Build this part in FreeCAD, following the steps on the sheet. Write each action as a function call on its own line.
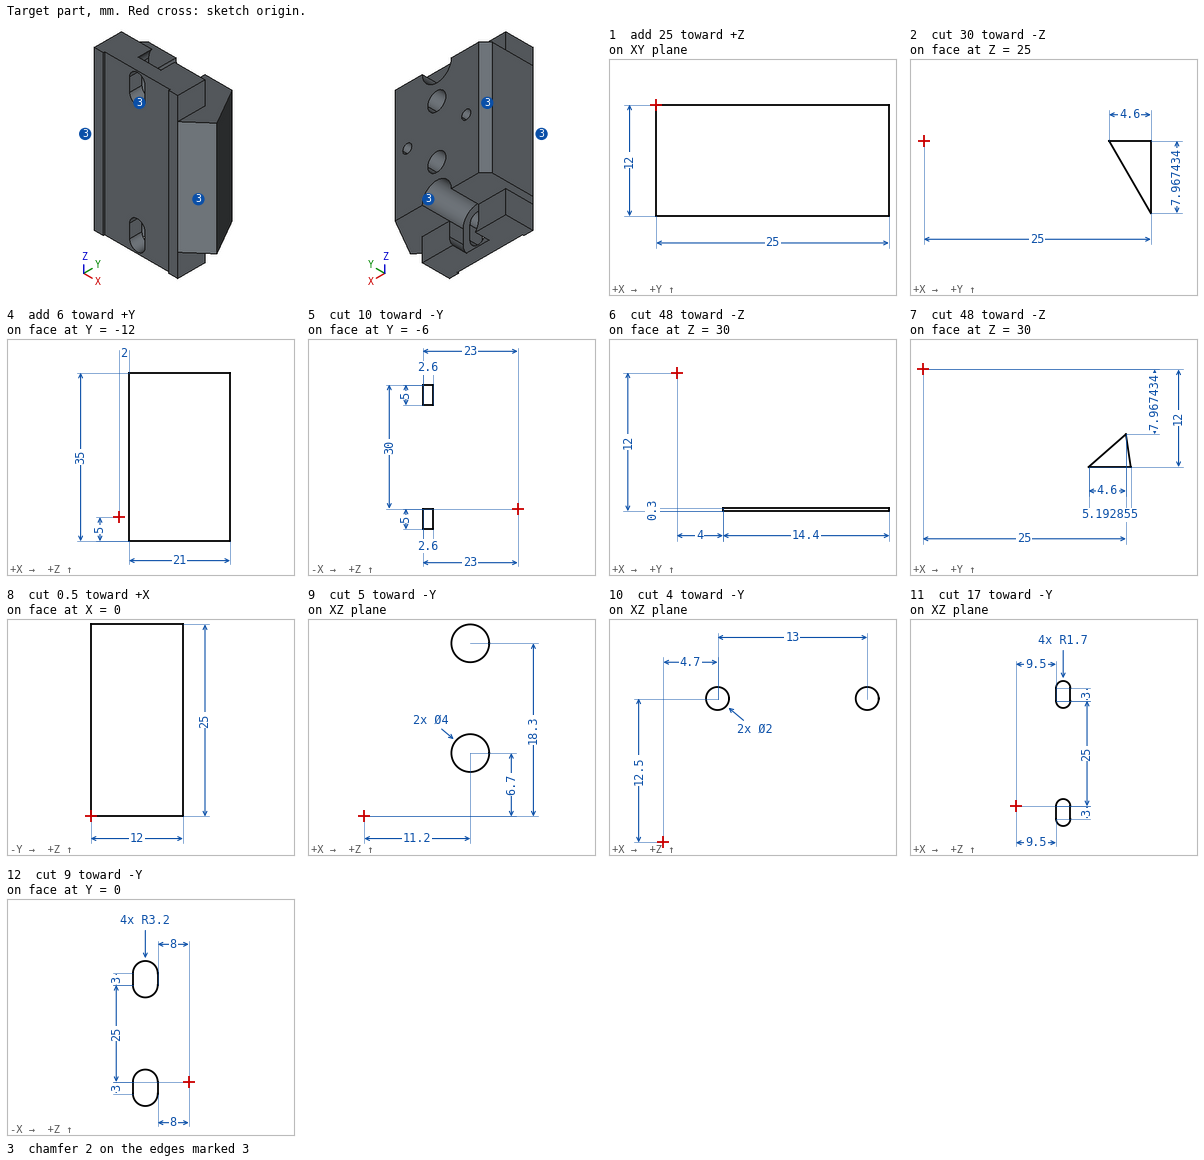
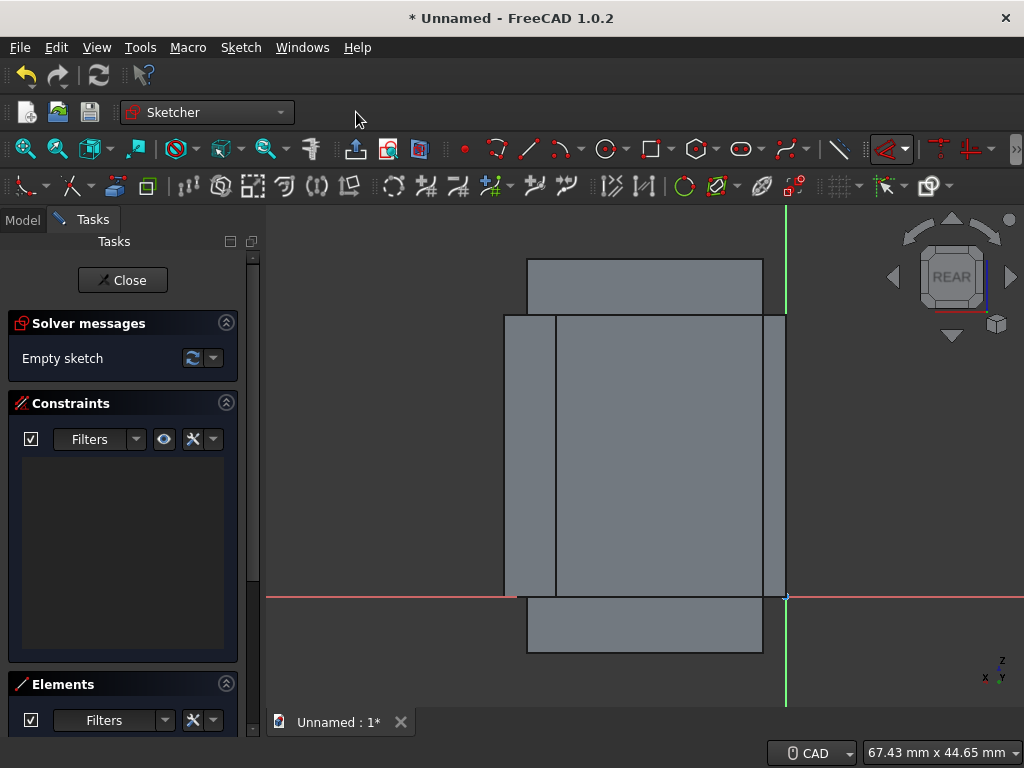
click(652, 150)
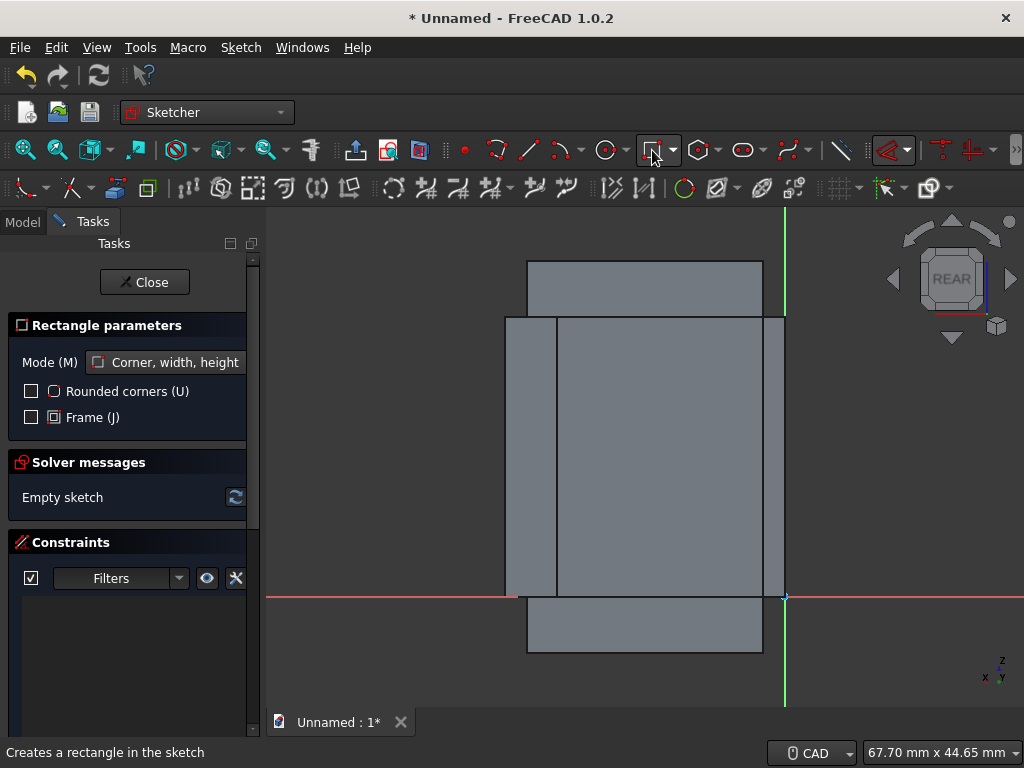
click(527, 261)
click(557, 317)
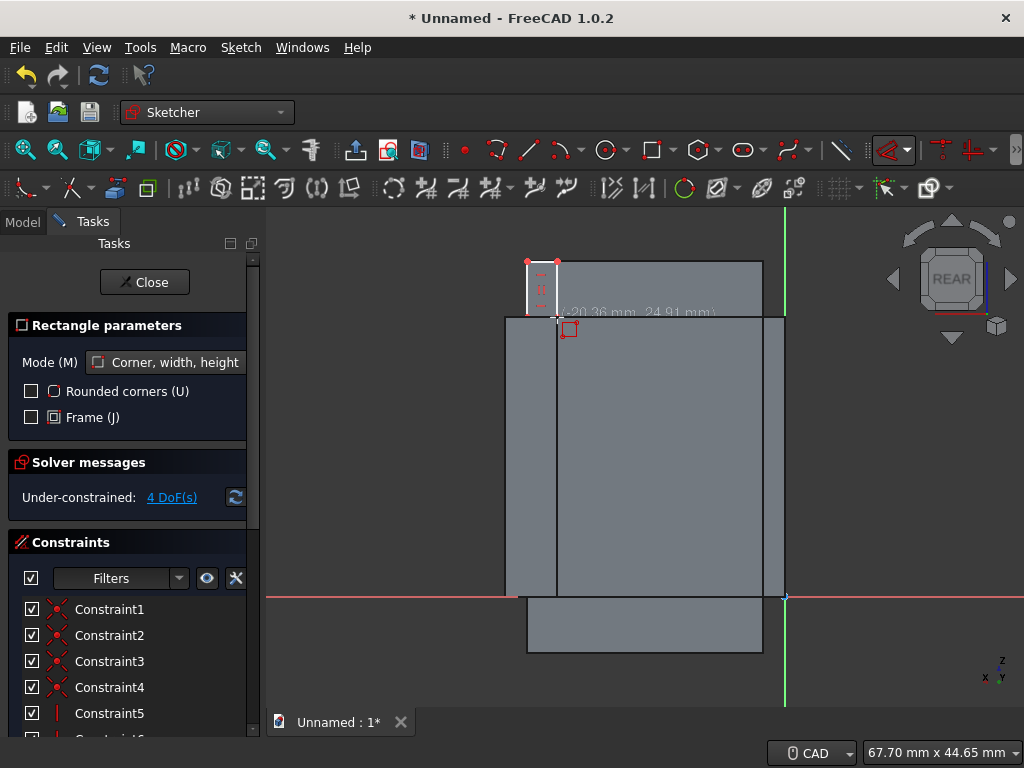
click(527, 597)
click(557, 653)
key(Escape)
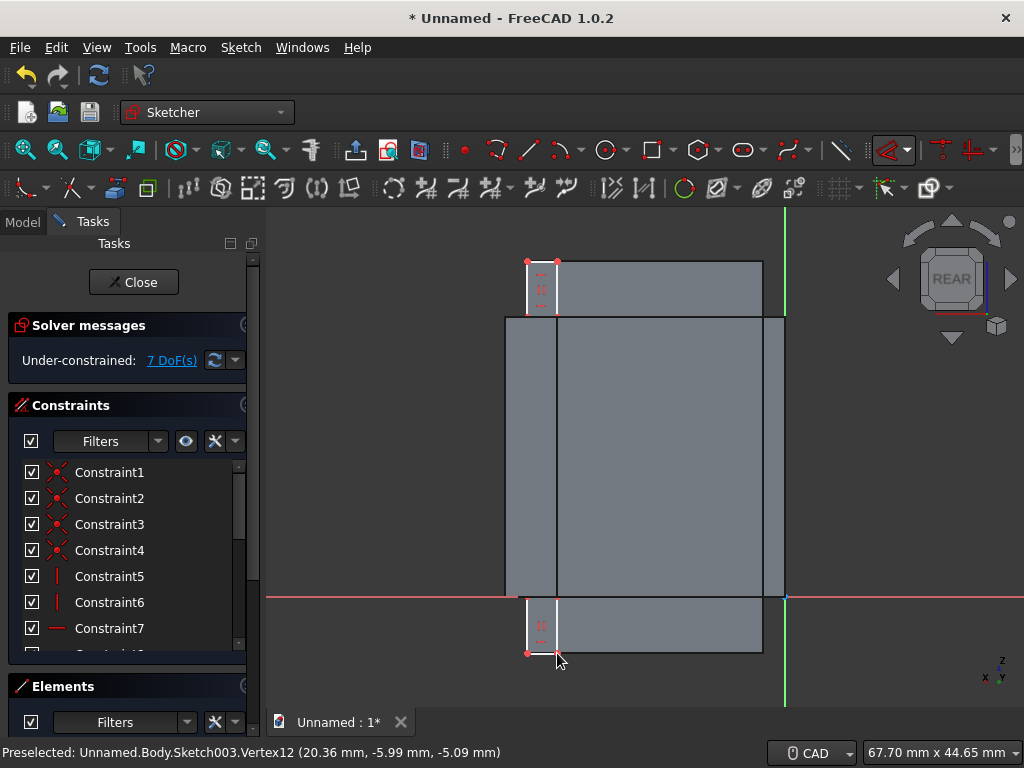
click(527, 279)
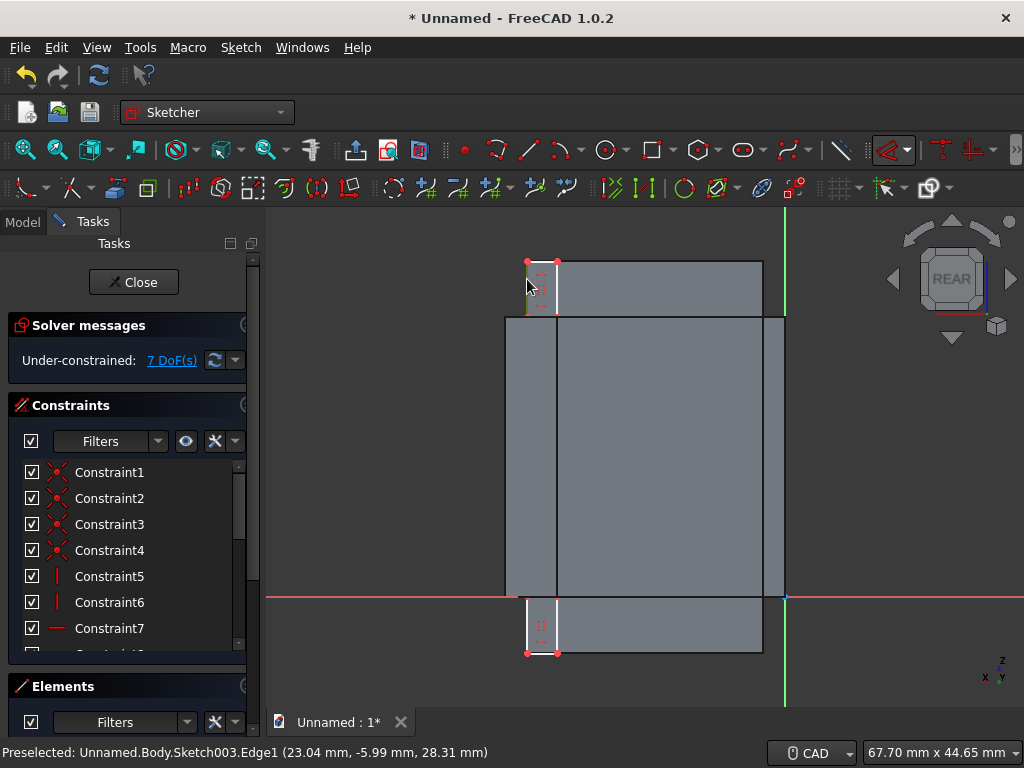
click(910, 150)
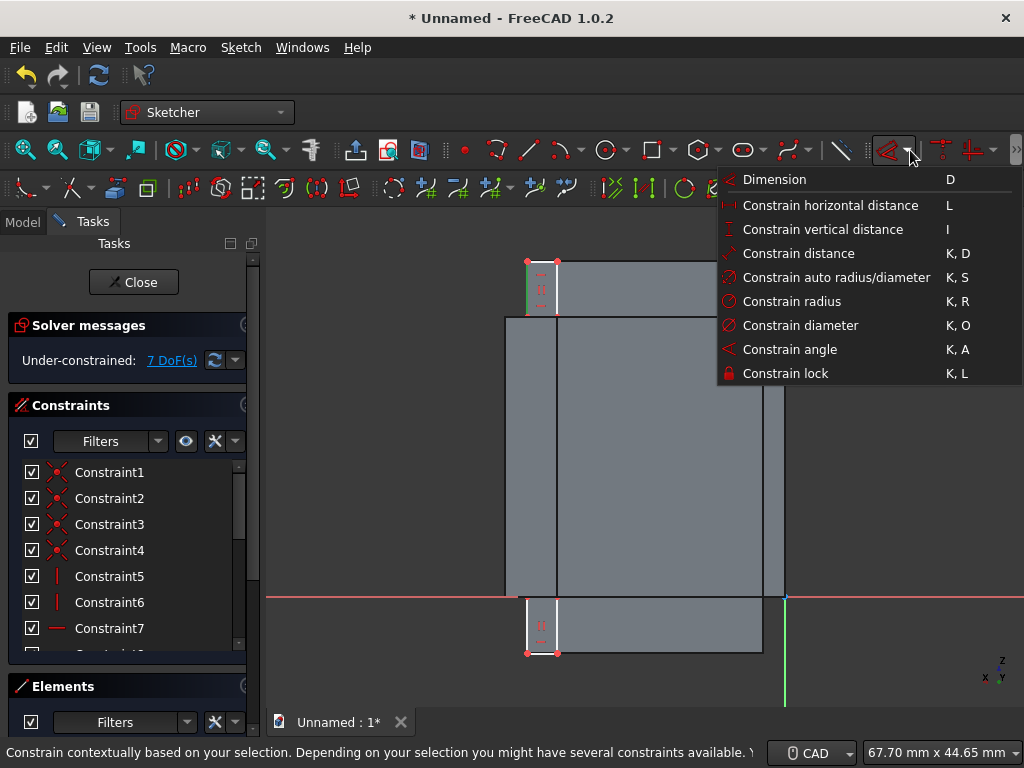
click(870, 229)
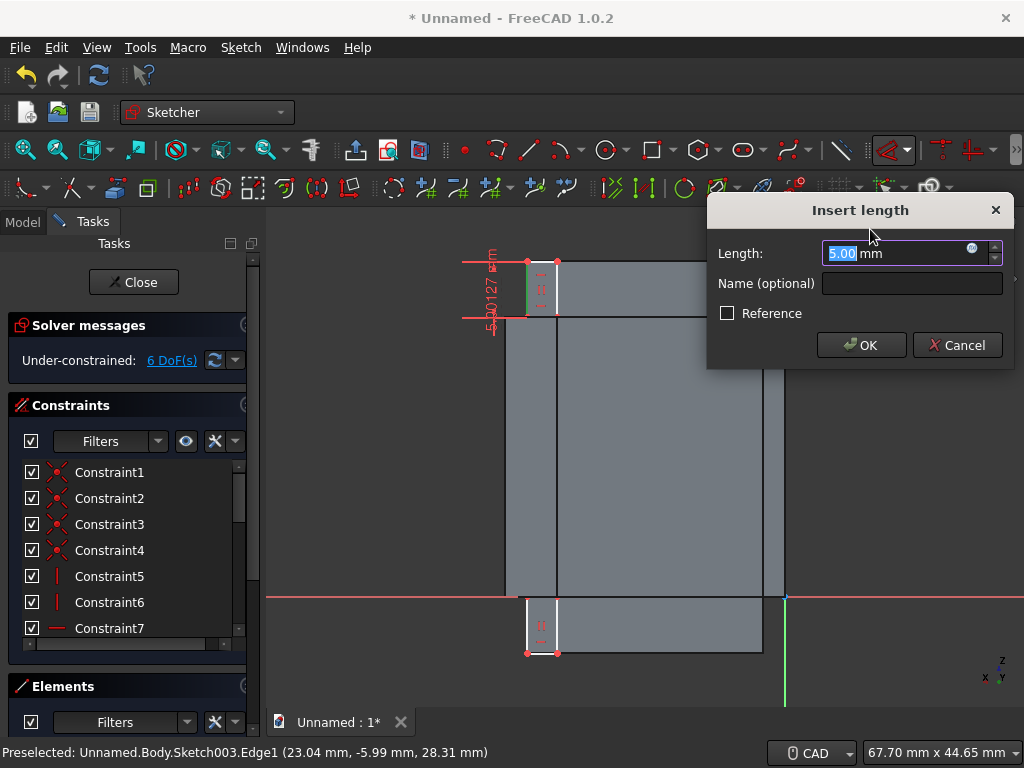
text(5)
key(Return)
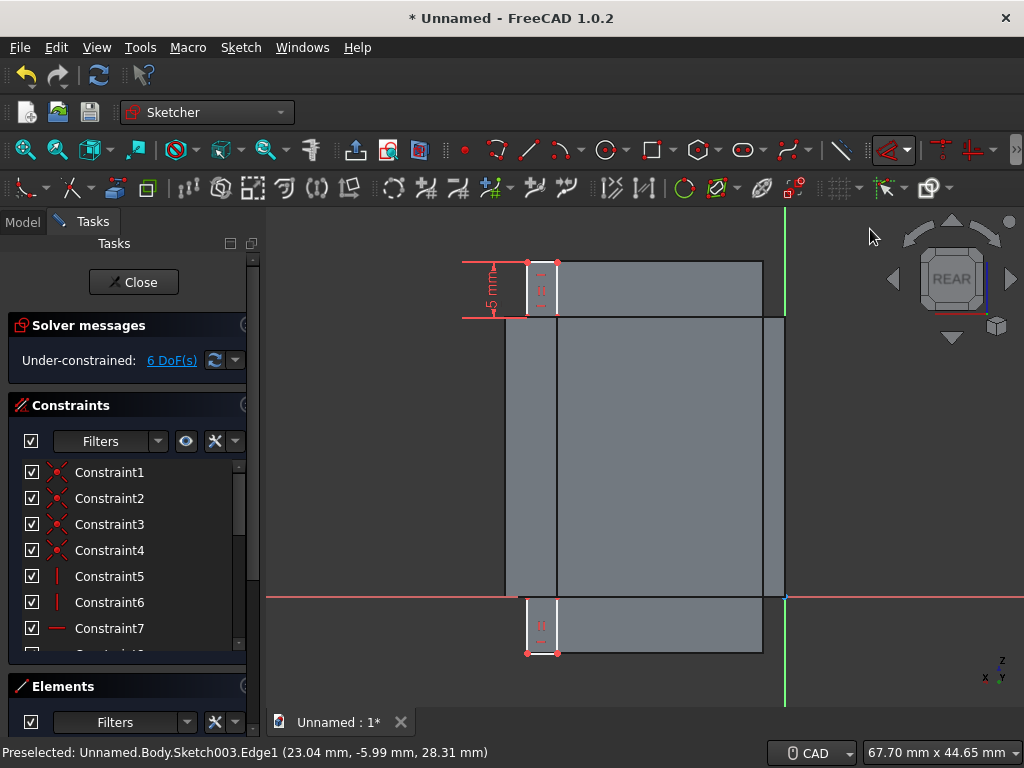
click(527, 614)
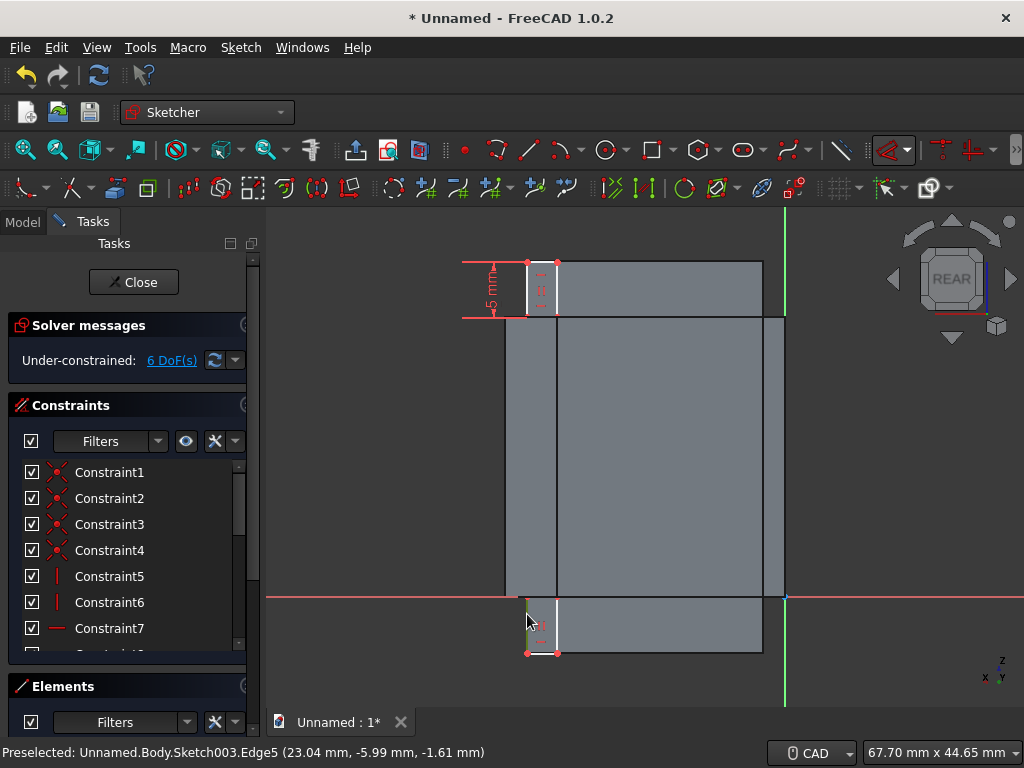
click(910, 150)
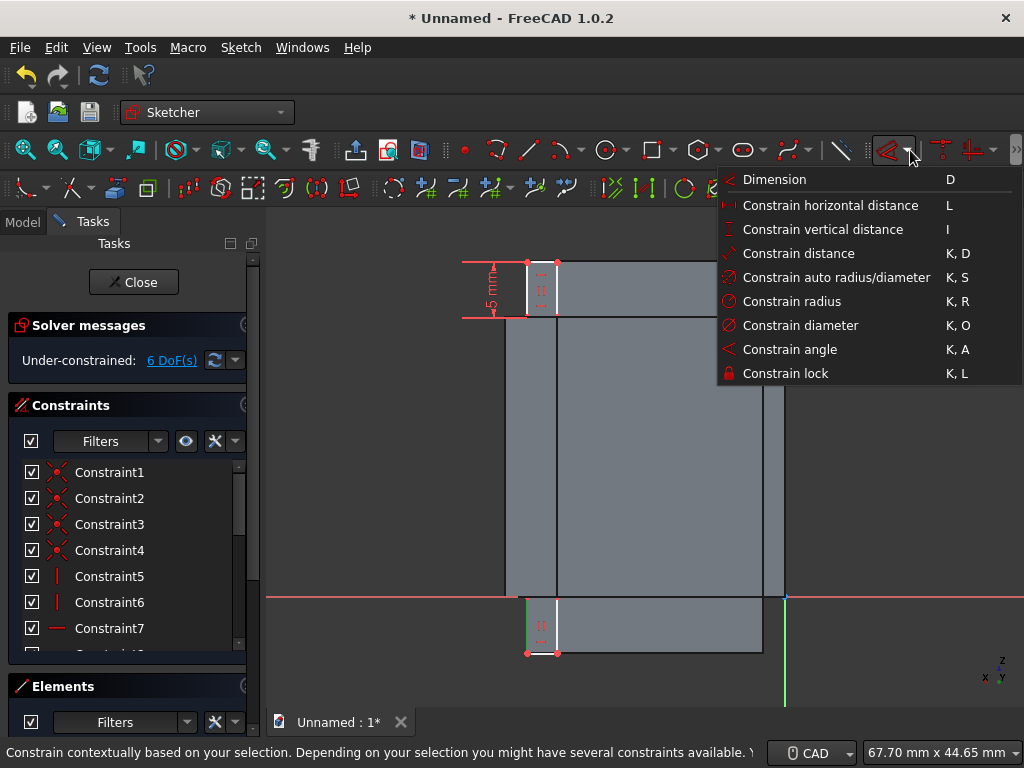
click(870, 229)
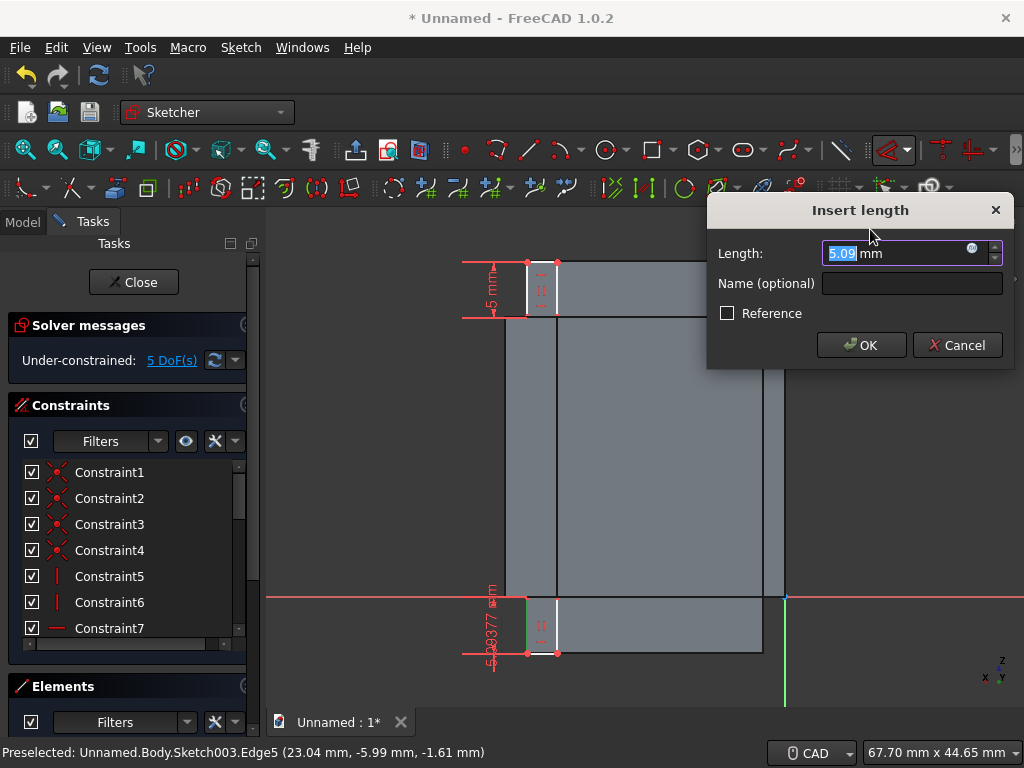
text(5)
key(Return)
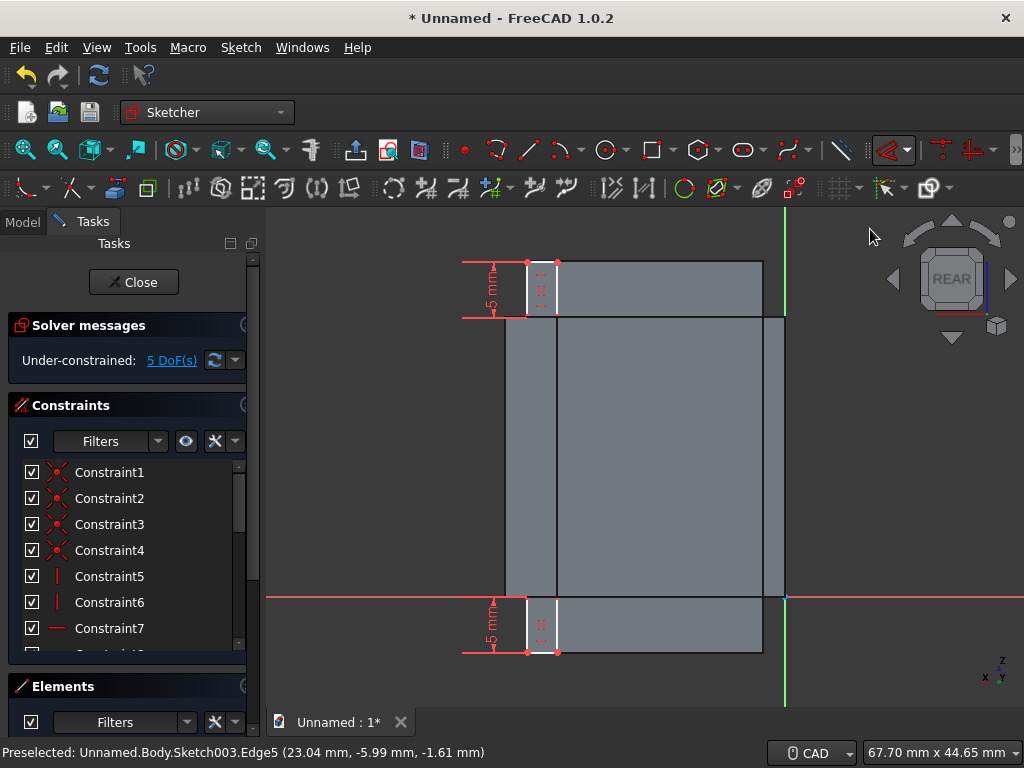
scroll(536, 318, up, 3)